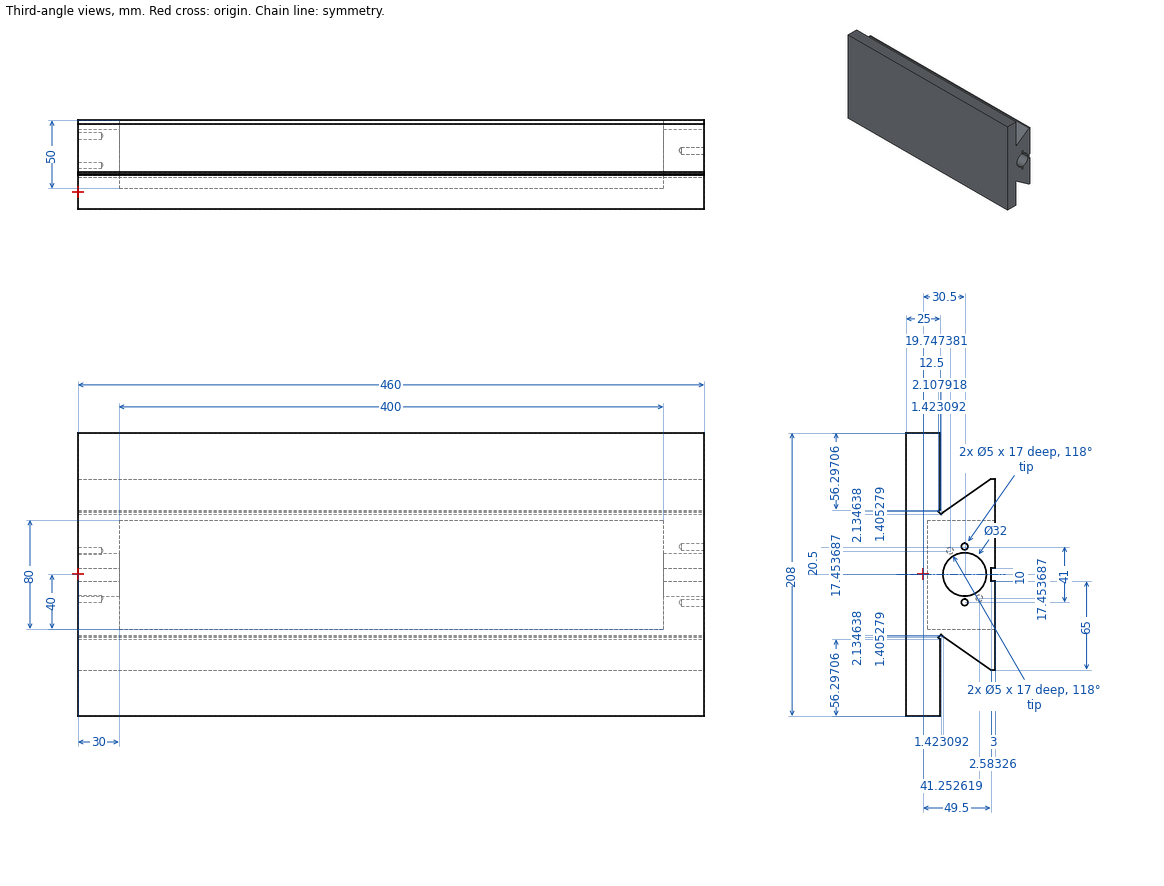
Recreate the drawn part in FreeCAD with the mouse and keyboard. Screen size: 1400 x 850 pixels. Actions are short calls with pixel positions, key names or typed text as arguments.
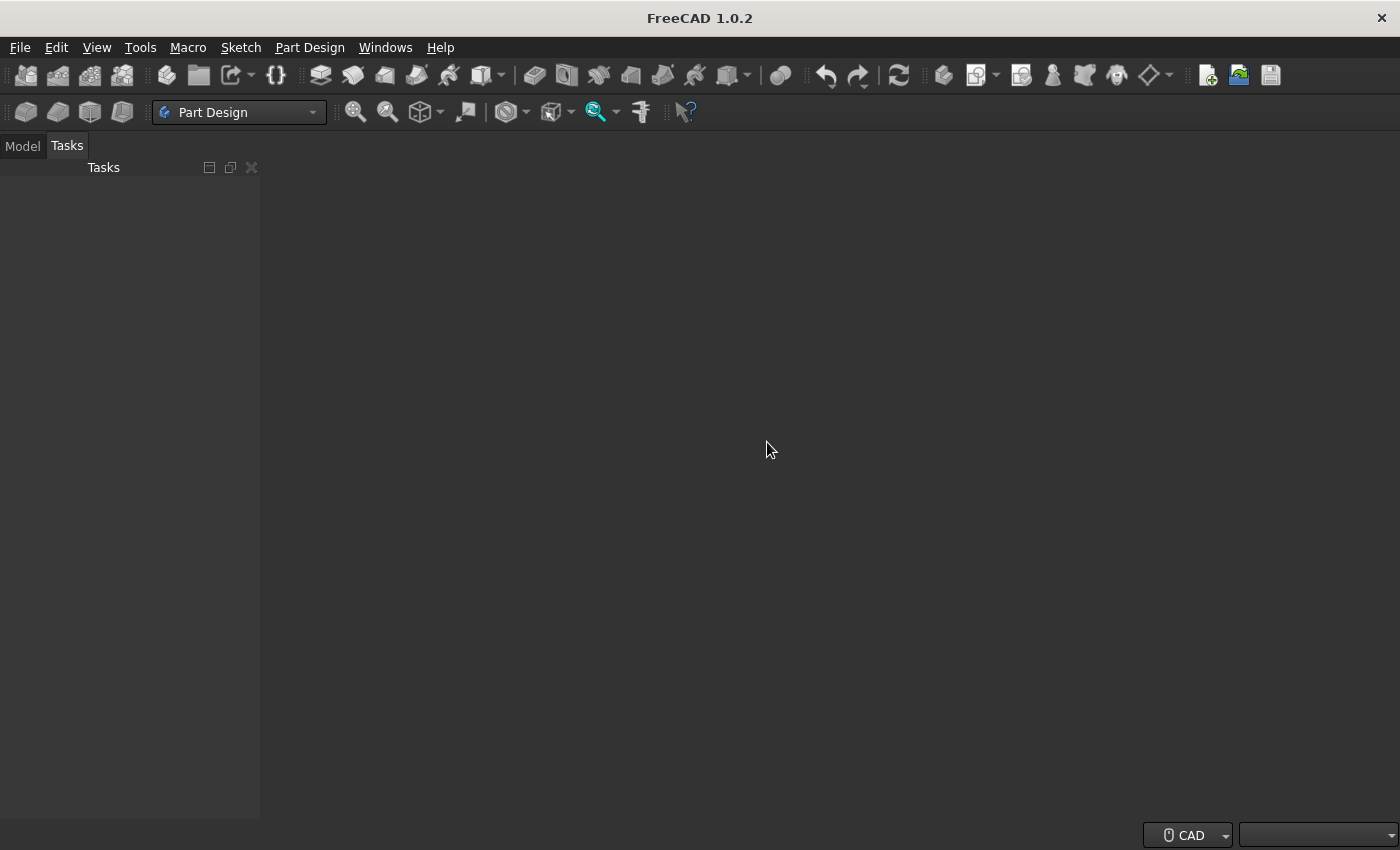
click(1208, 76)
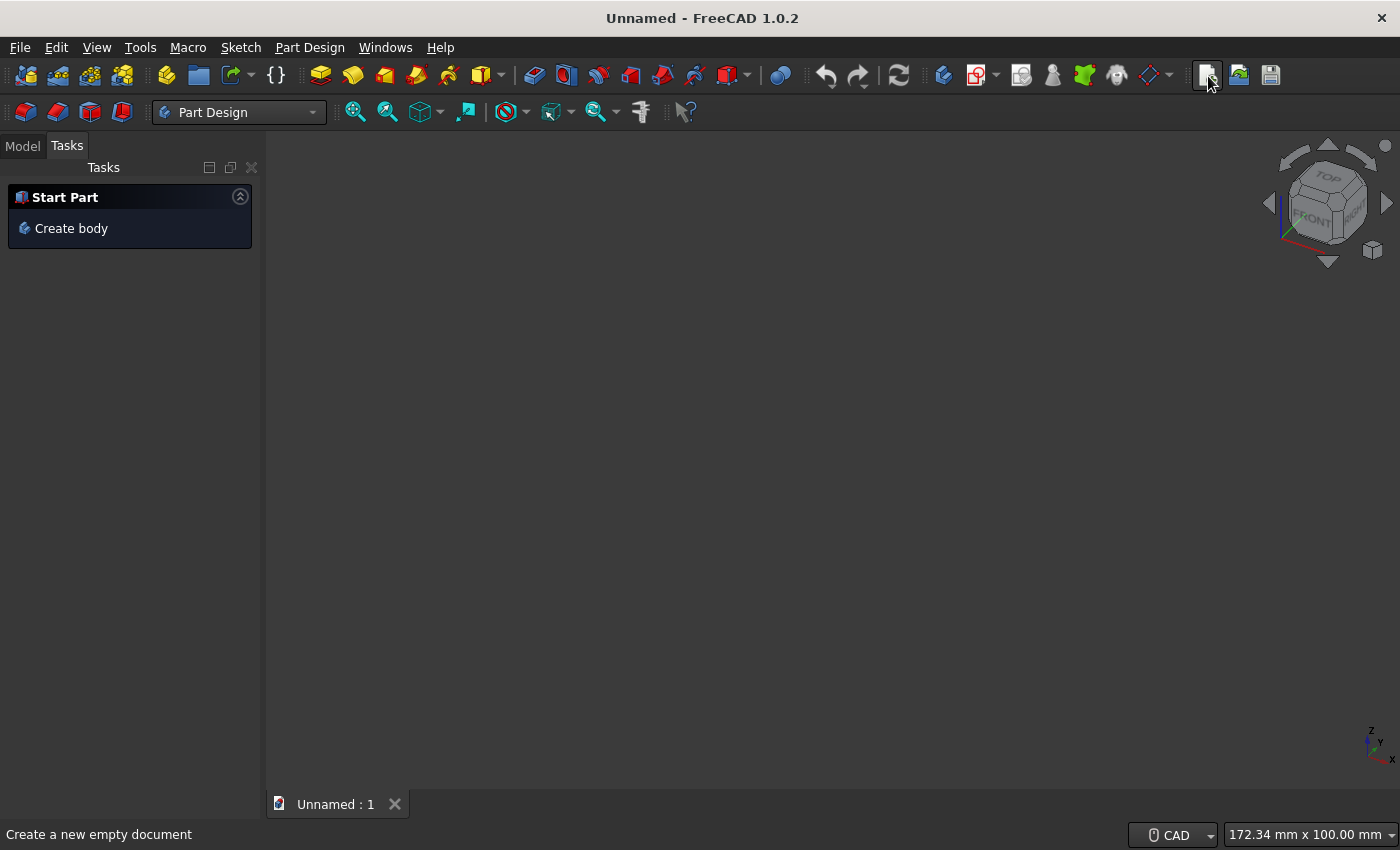
click(976, 76)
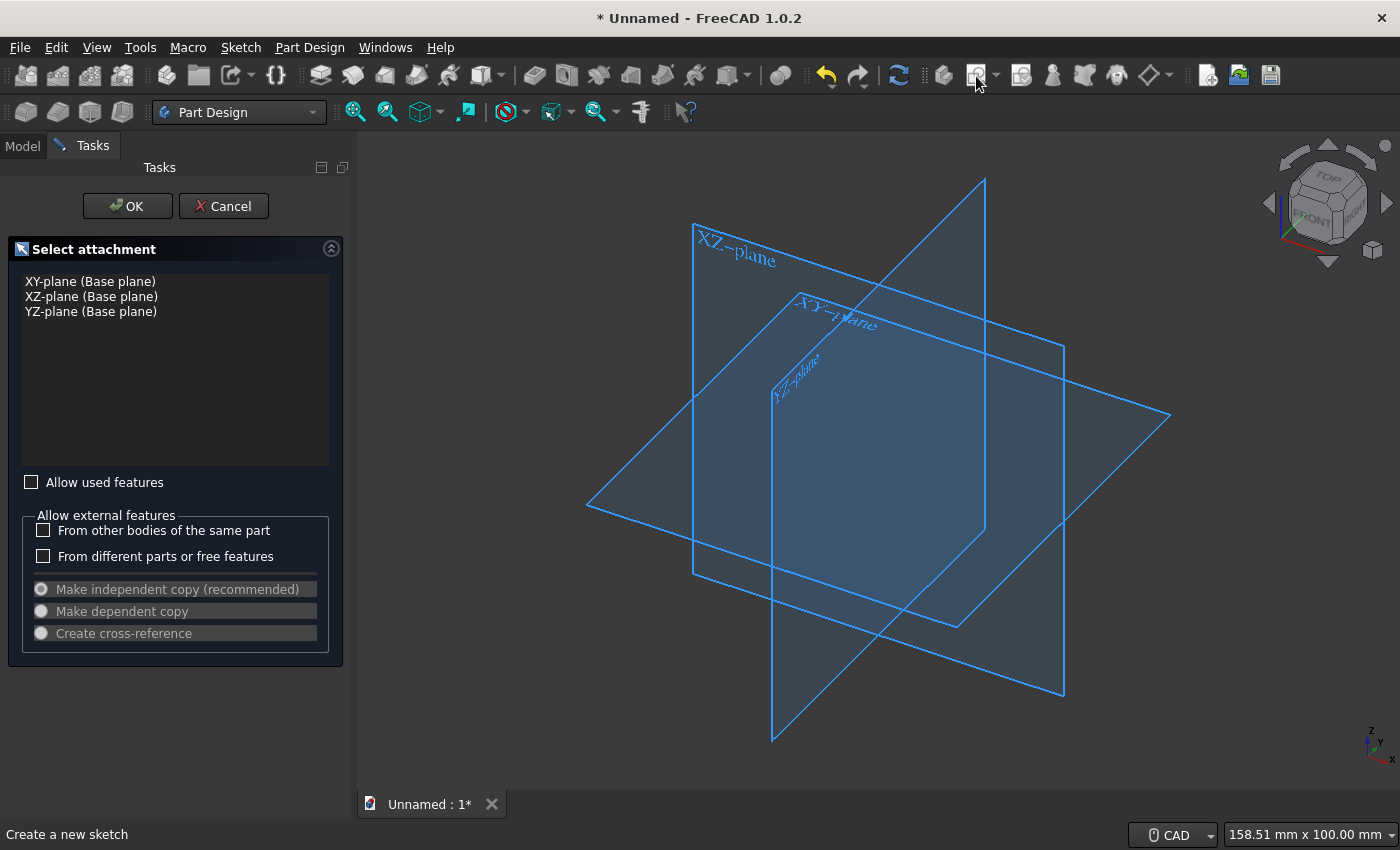
click(82, 312)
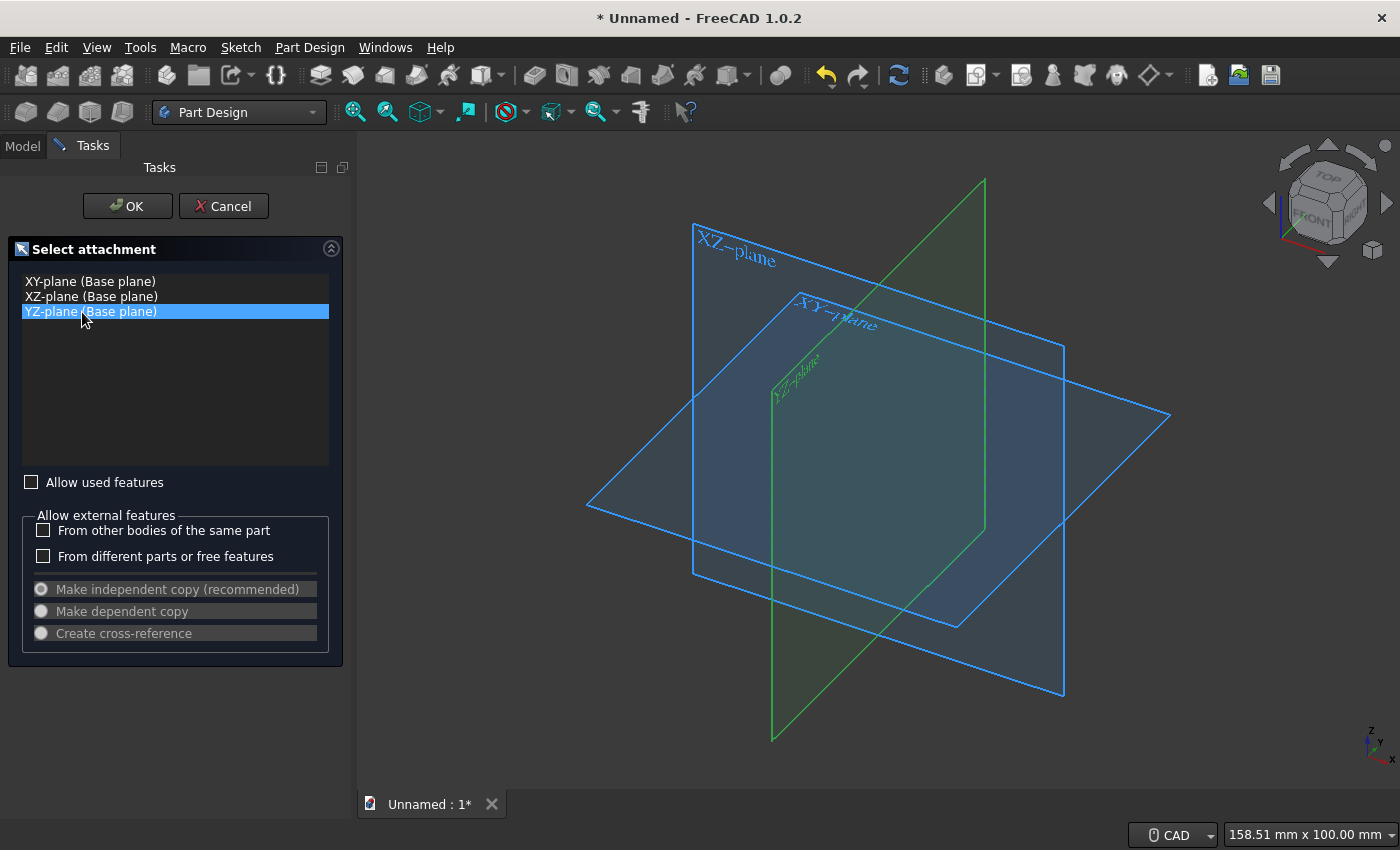
click(128, 206)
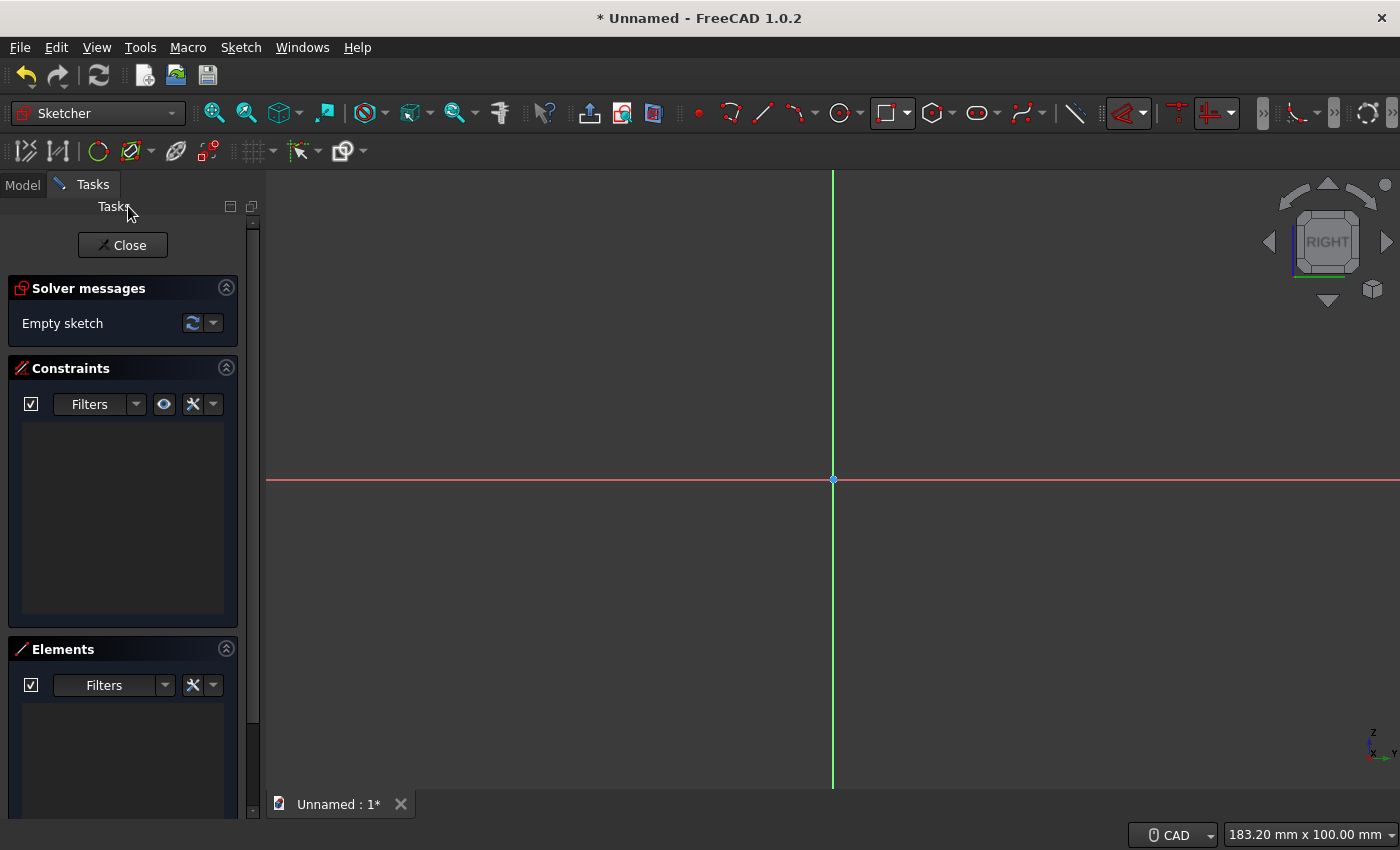
scroll(682, 480, down, 6)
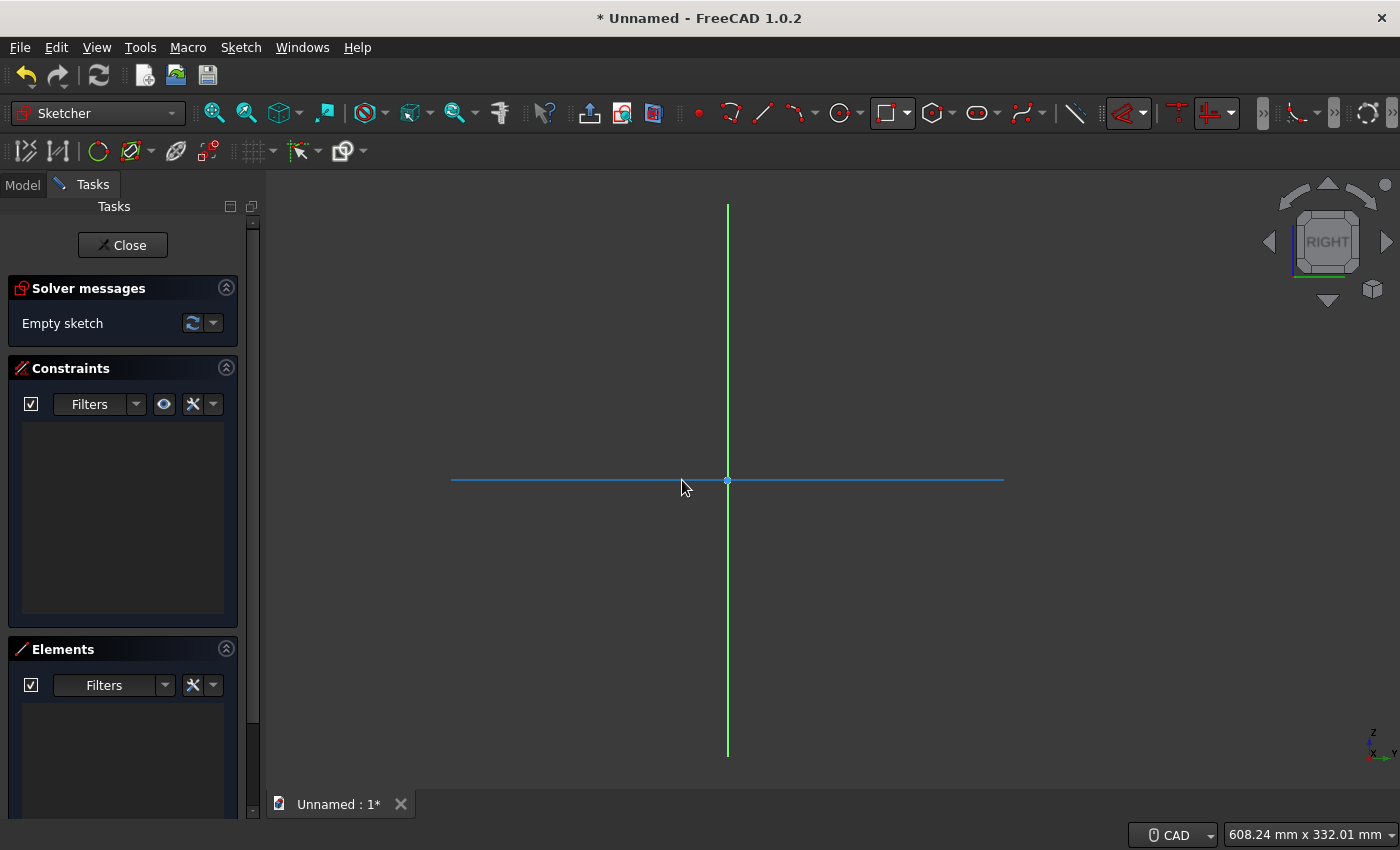
click(732, 114)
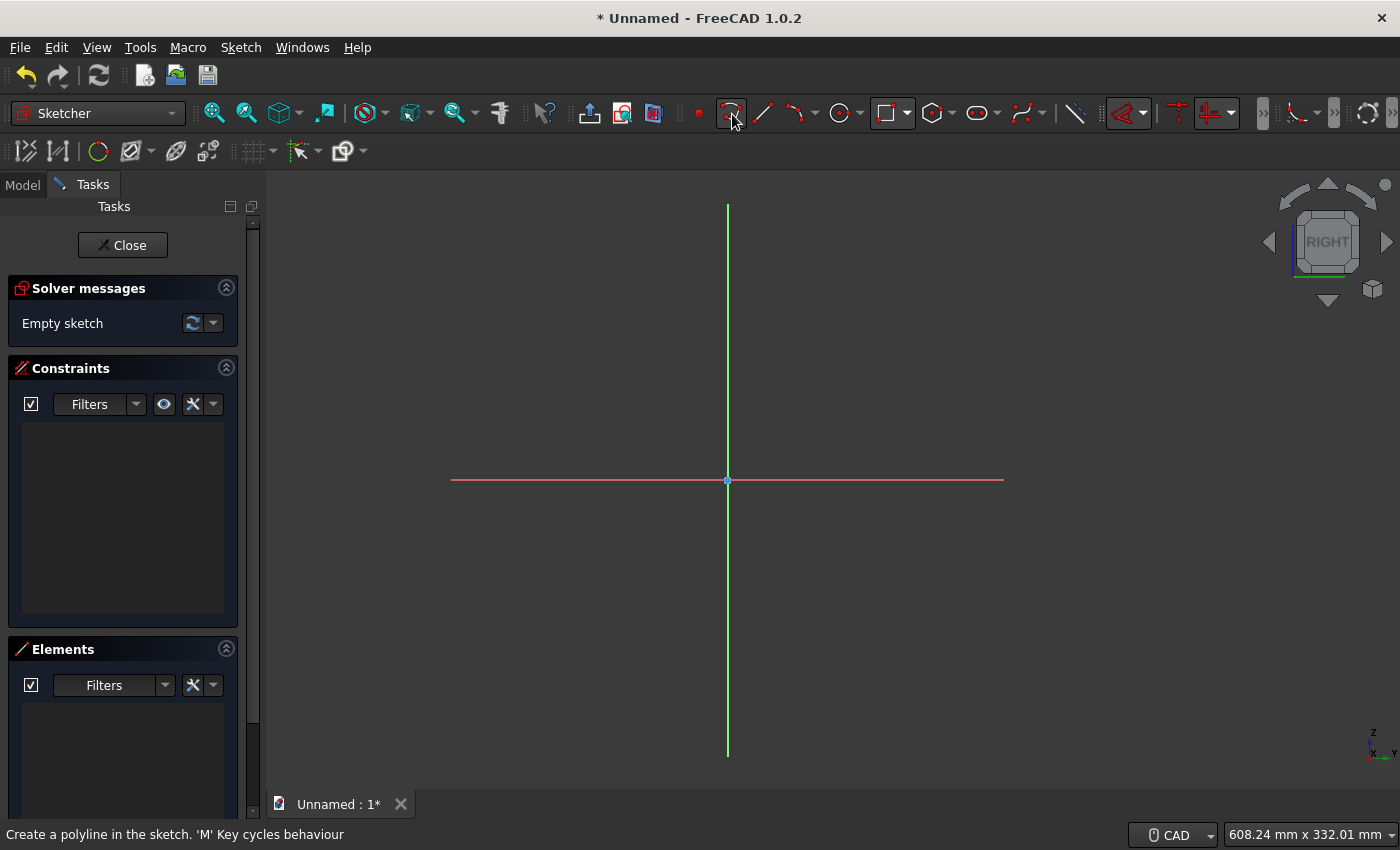
click(752, 563)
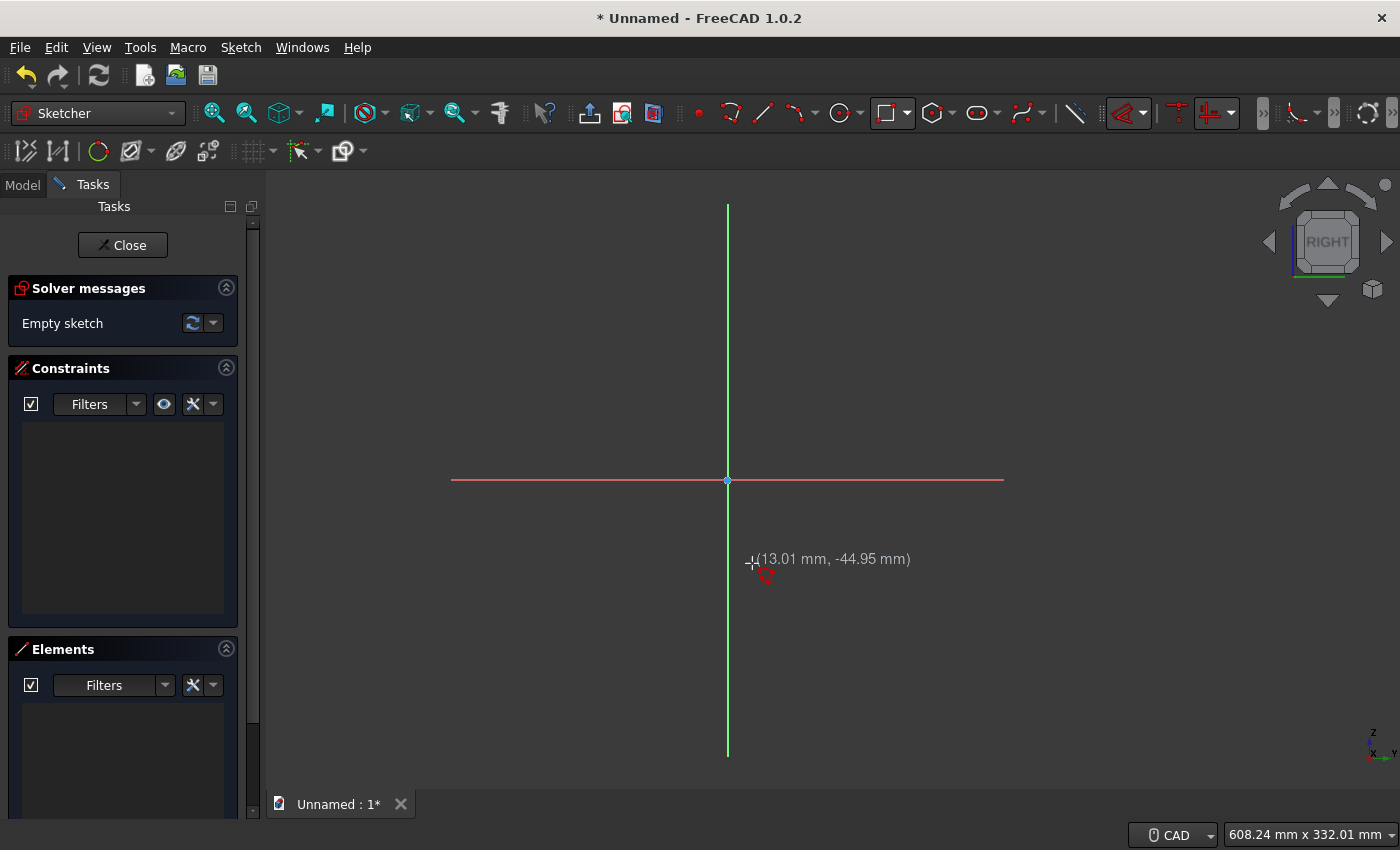
scroll(755, 565, up, 8)